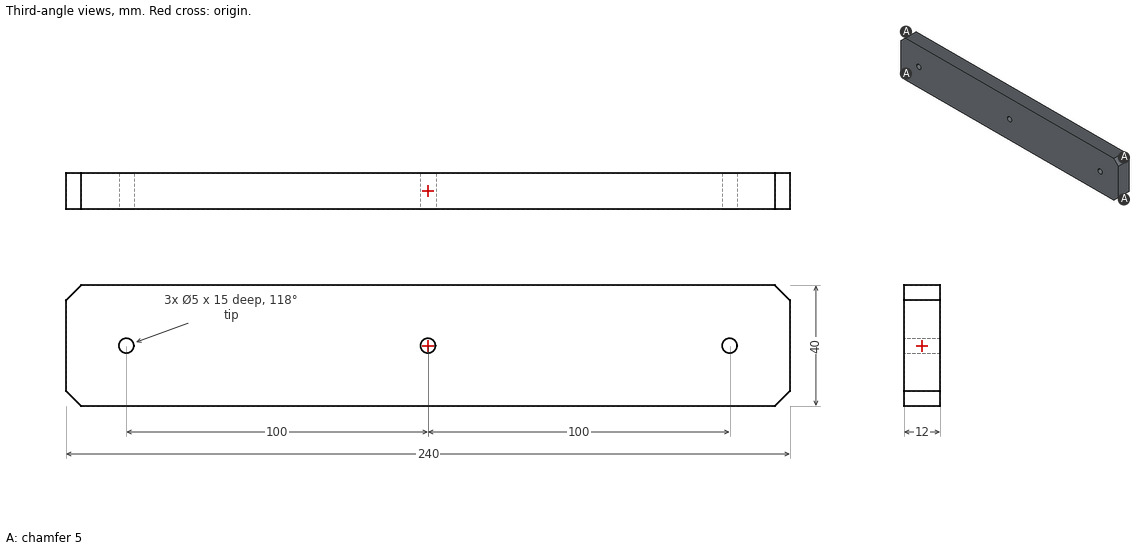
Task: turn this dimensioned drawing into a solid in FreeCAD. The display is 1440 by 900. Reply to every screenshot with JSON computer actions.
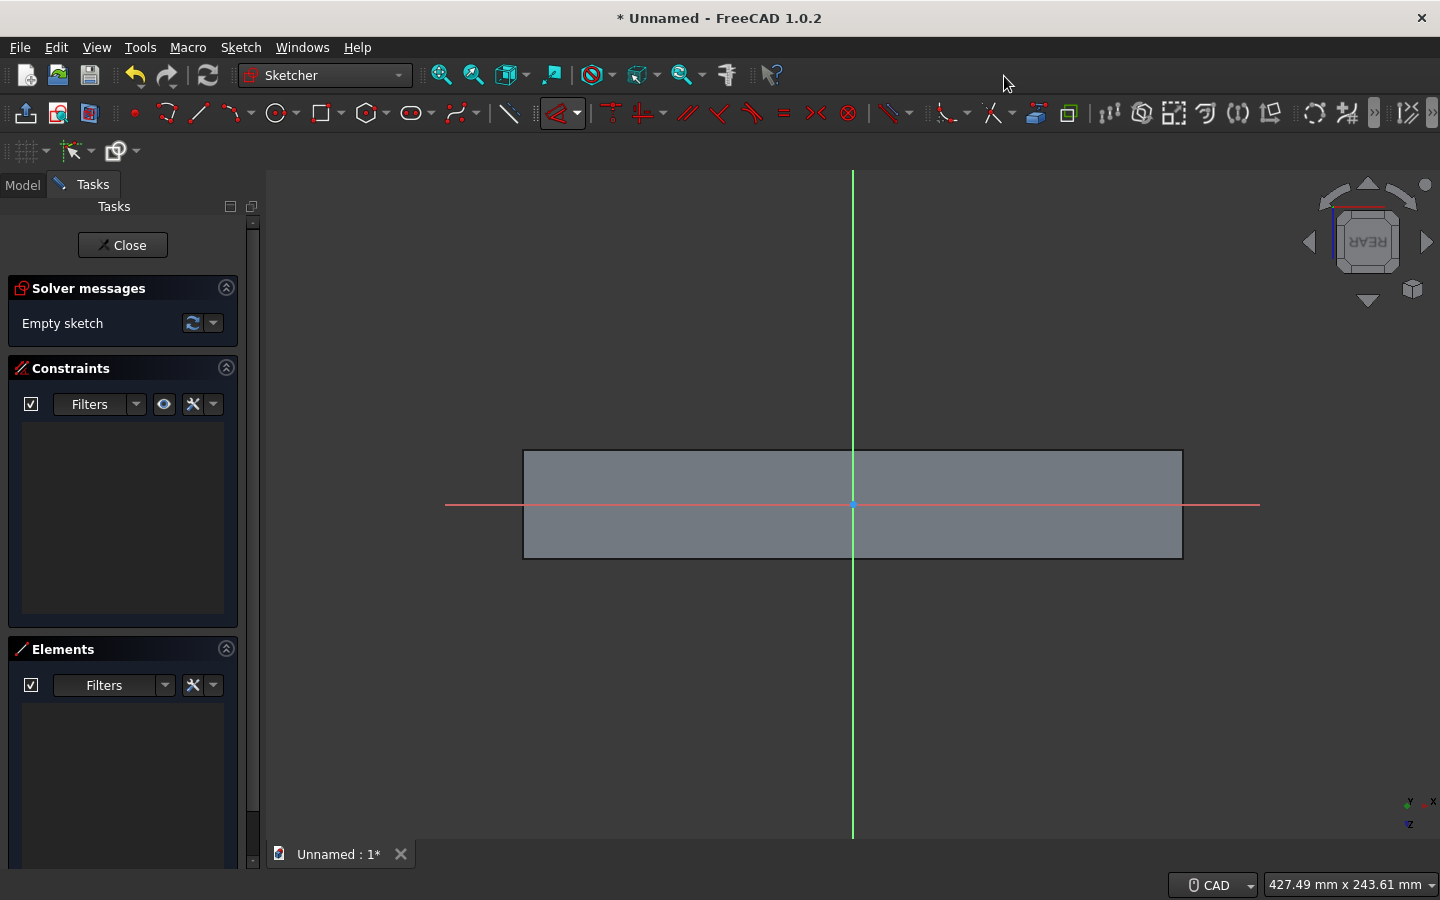
{"action": "left_click", "coordinate": [276, 114]}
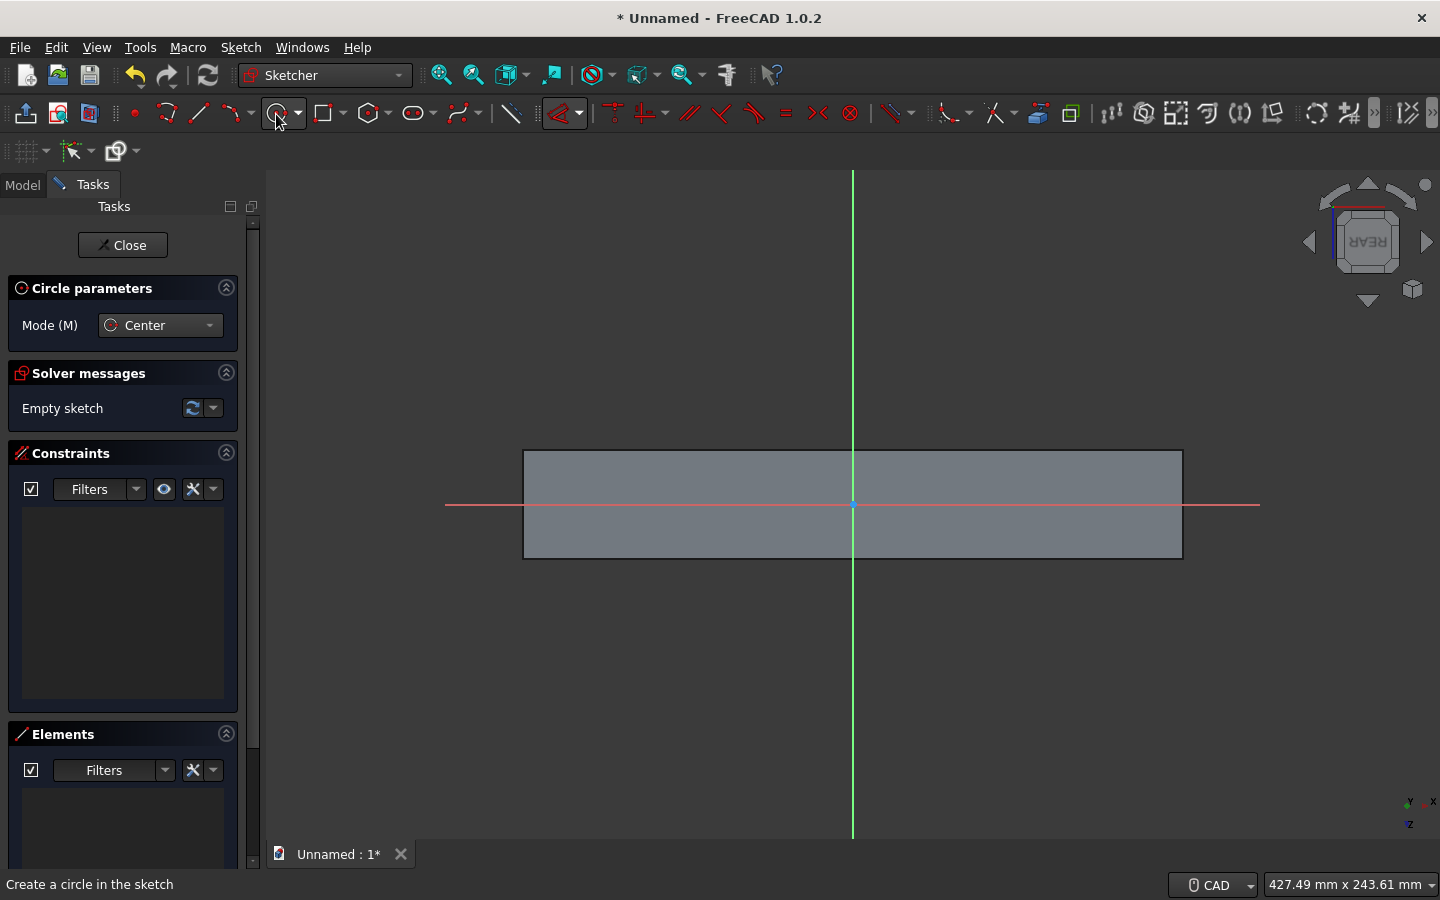
{"action": "scroll", "coordinate": [578, 505], "scroll_direction": "up", "scroll_amount": 6}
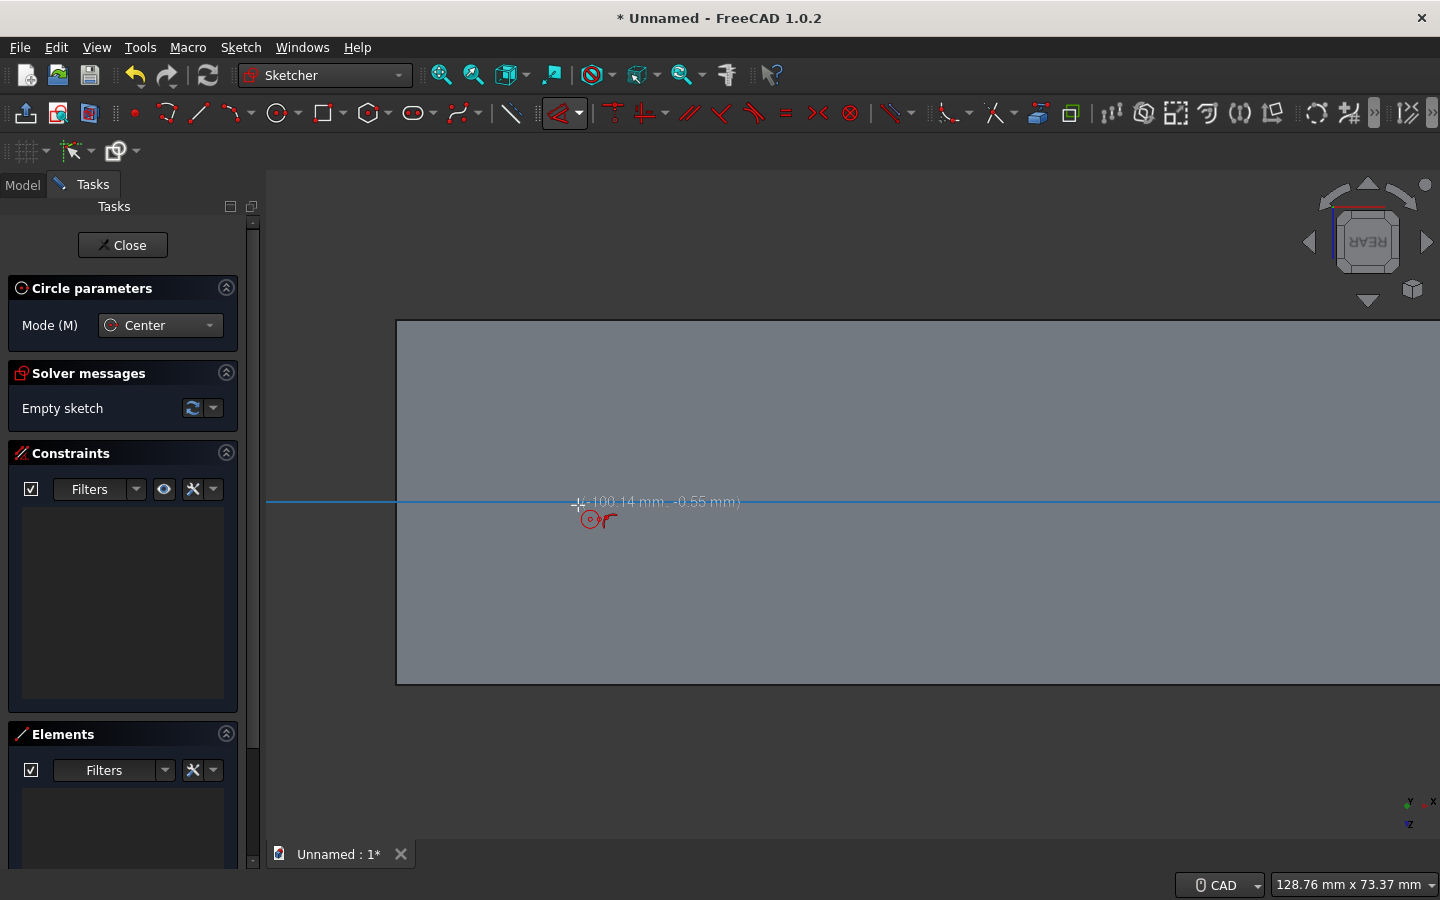
{"action": "left_click", "coordinate": [579, 502]}
{"action": "left_click", "coordinate": [595, 486]}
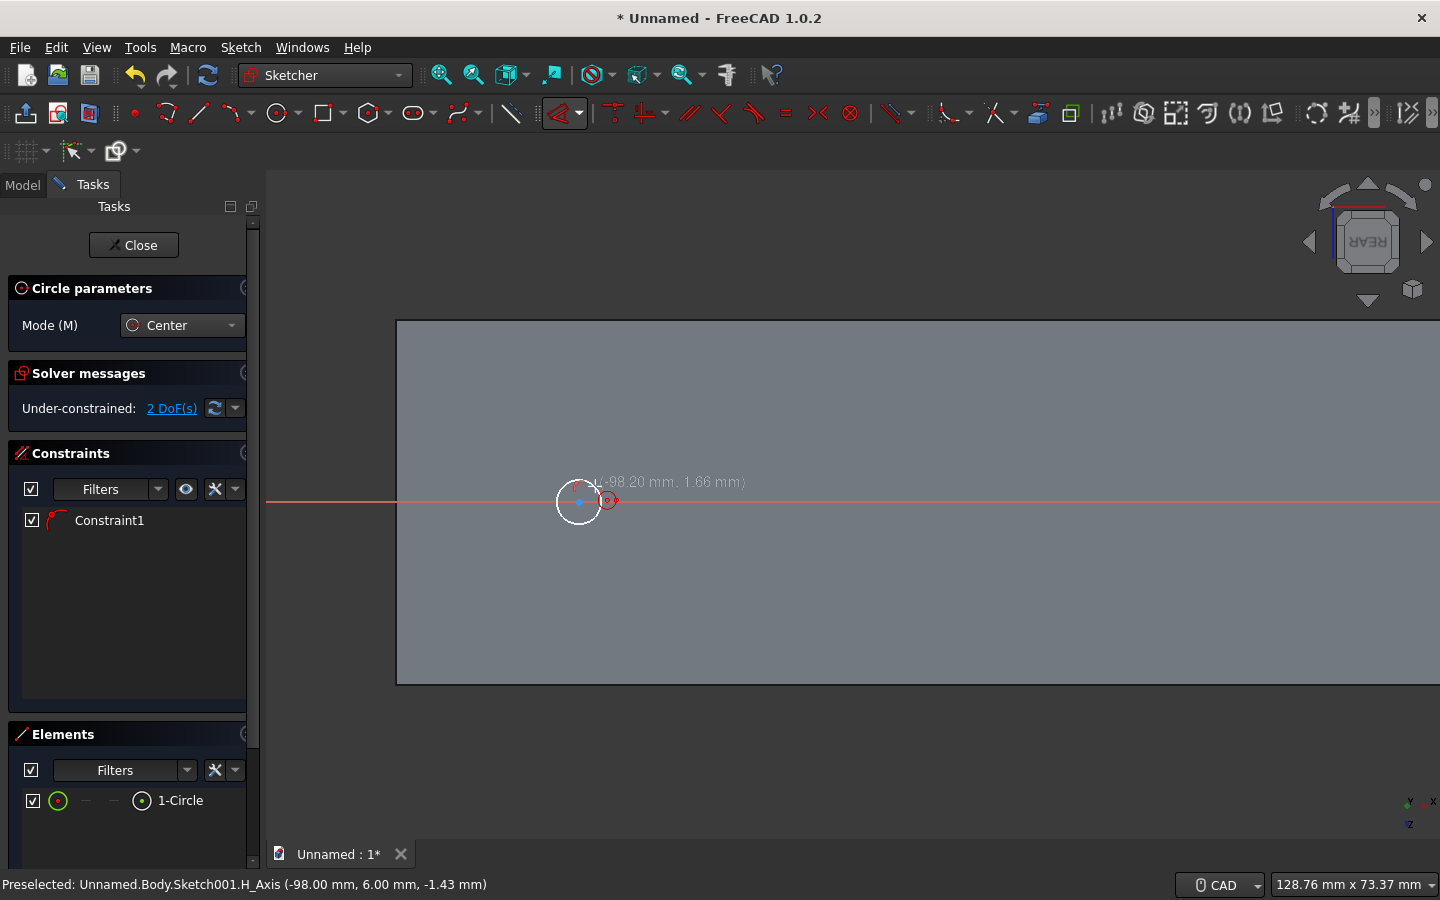
{"action": "scroll", "coordinate": [374, 506], "scroll_direction": "down", "scroll_amount": 5}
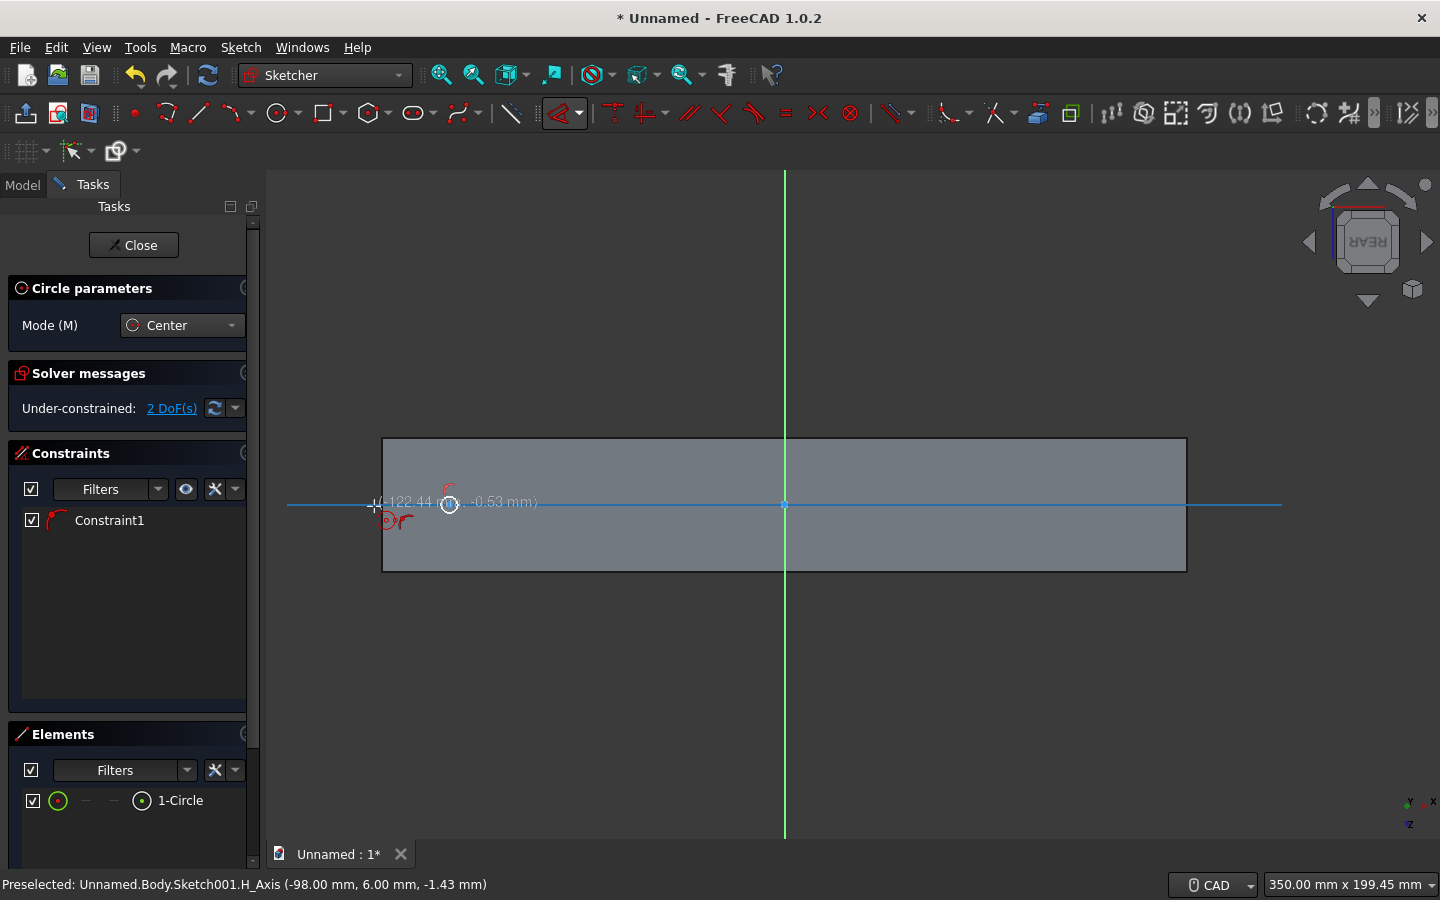
{"action": "scroll", "coordinate": [785, 505], "scroll_direction": "up", "scroll_amount": 5}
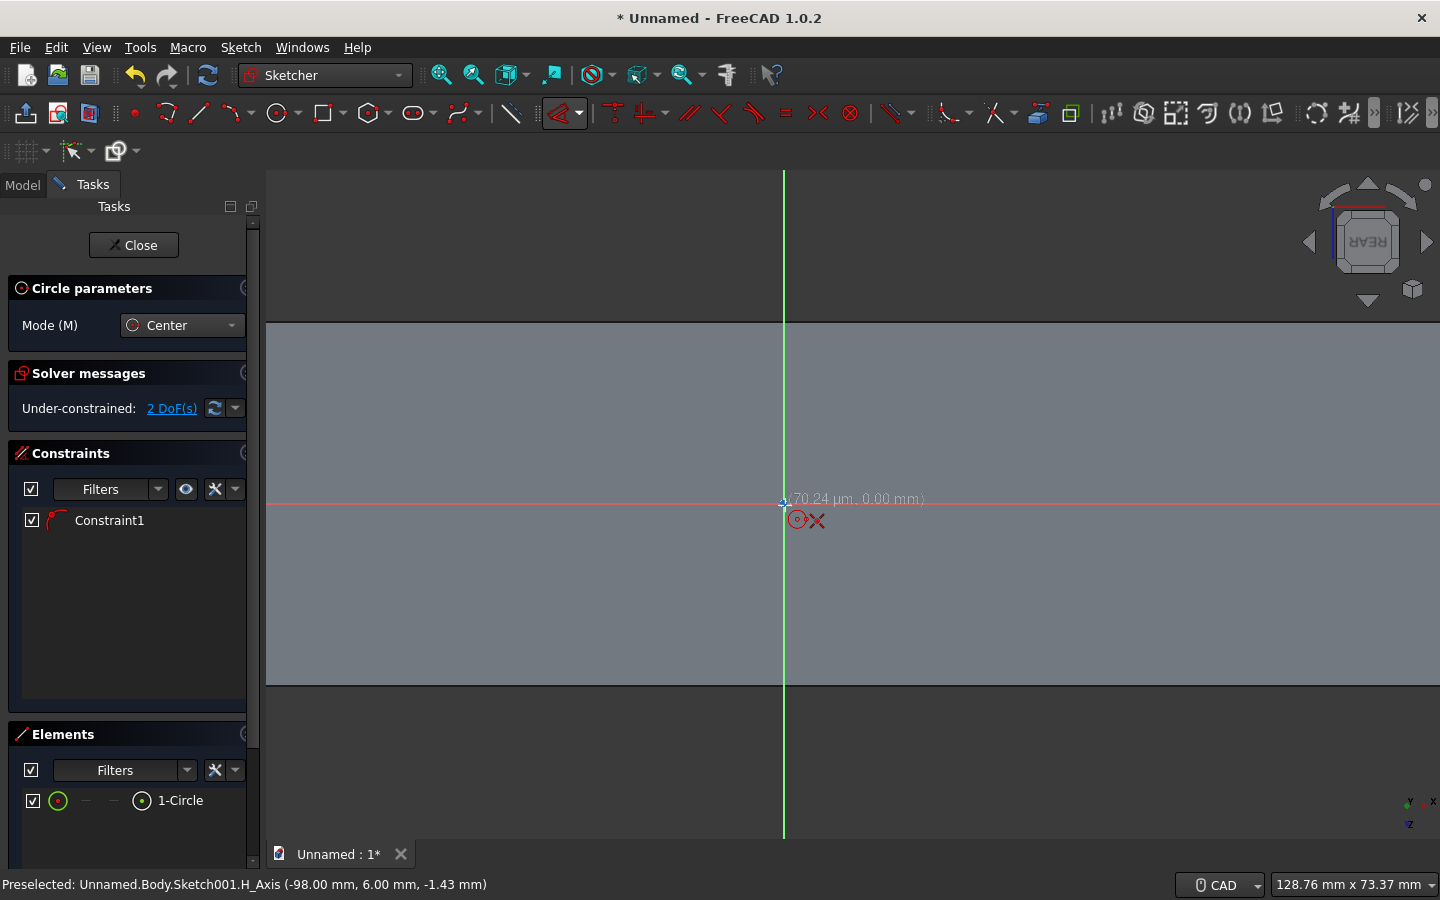
{"action": "left_click", "coordinate": [784, 504]}
{"action": "left_click", "coordinate": [800, 488]}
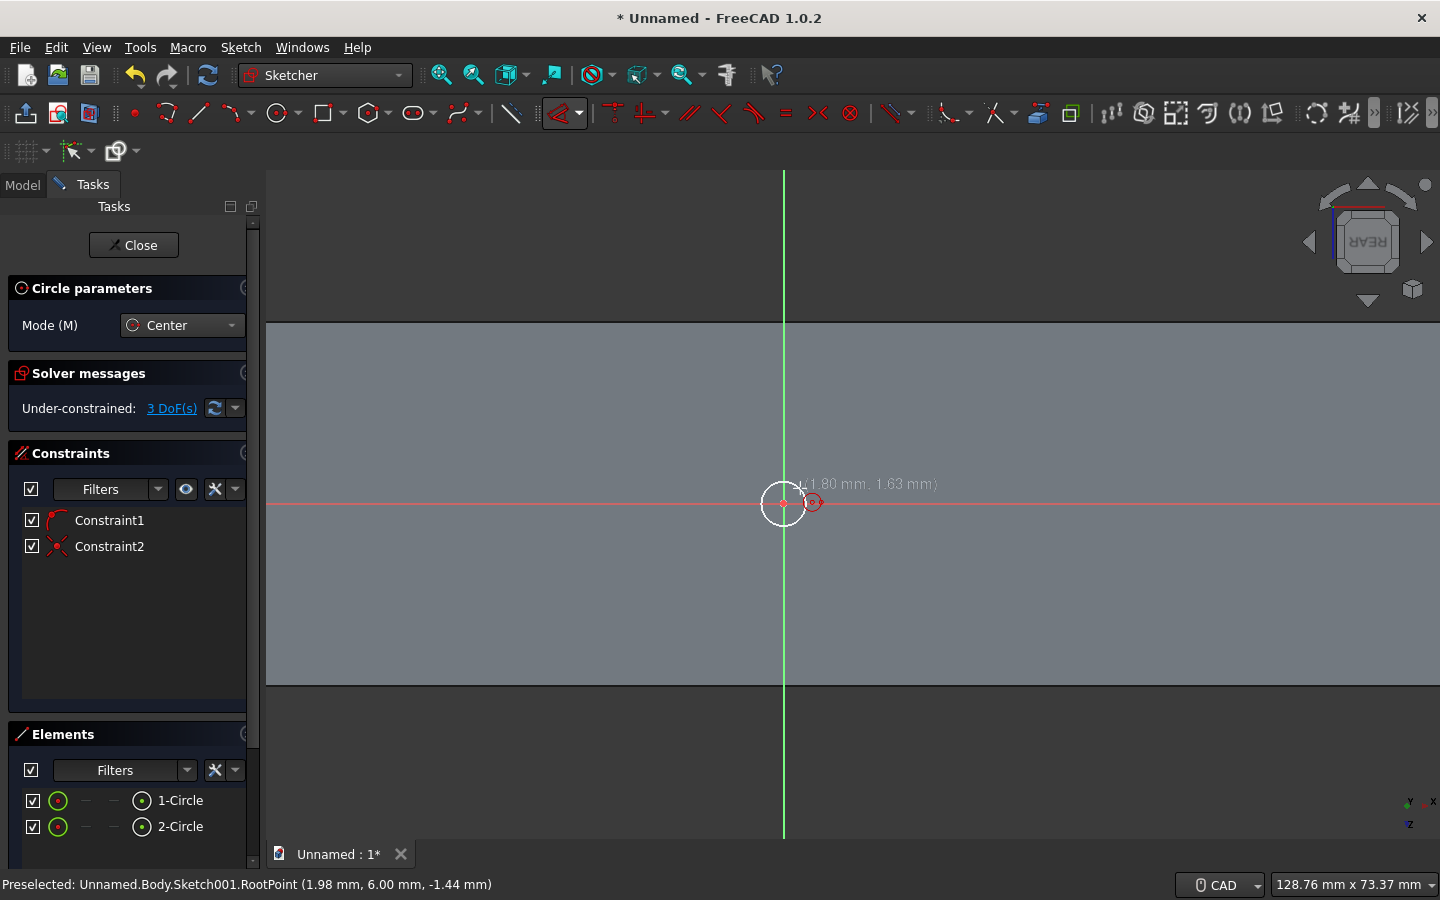
{"action": "scroll", "coordinate": [785, 505], "scroll_direction": "down", "scroll_amount": 5}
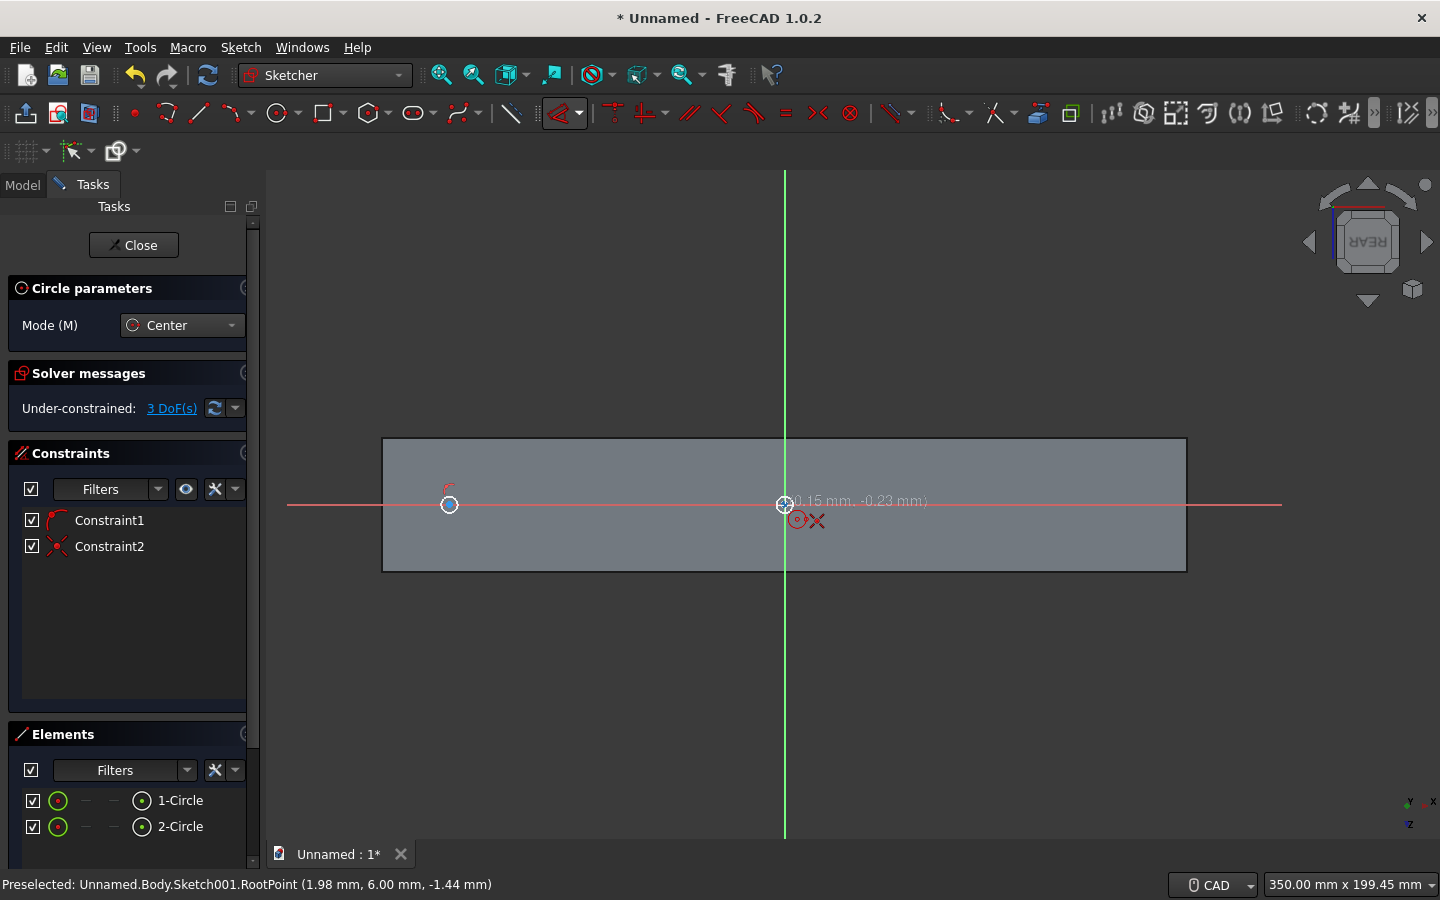
{"action": "scroll", "coordinate": [1120, 505], "scroll_direction": "up", "scroll_amount": 5}